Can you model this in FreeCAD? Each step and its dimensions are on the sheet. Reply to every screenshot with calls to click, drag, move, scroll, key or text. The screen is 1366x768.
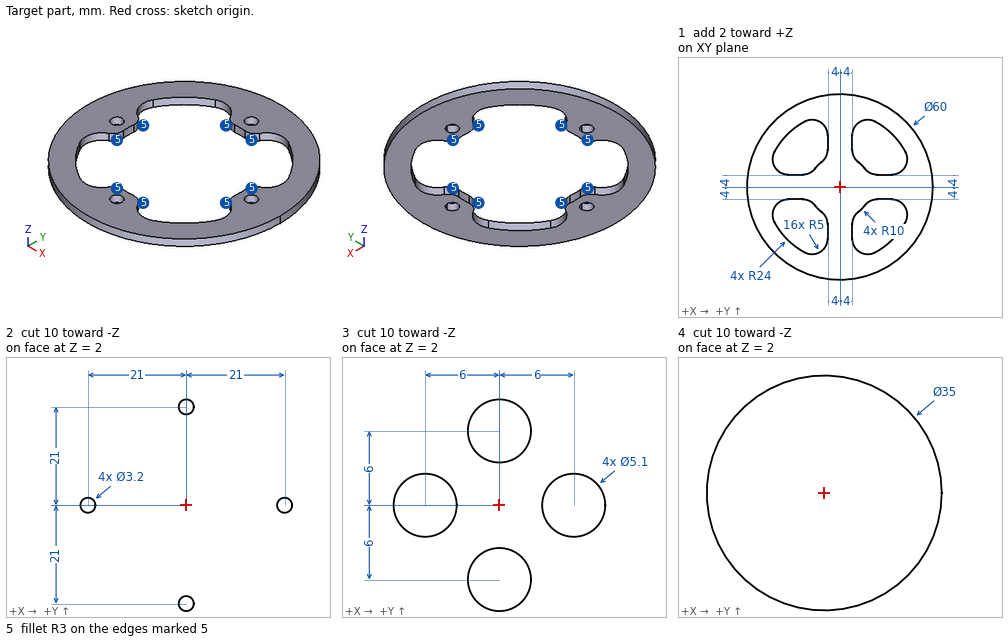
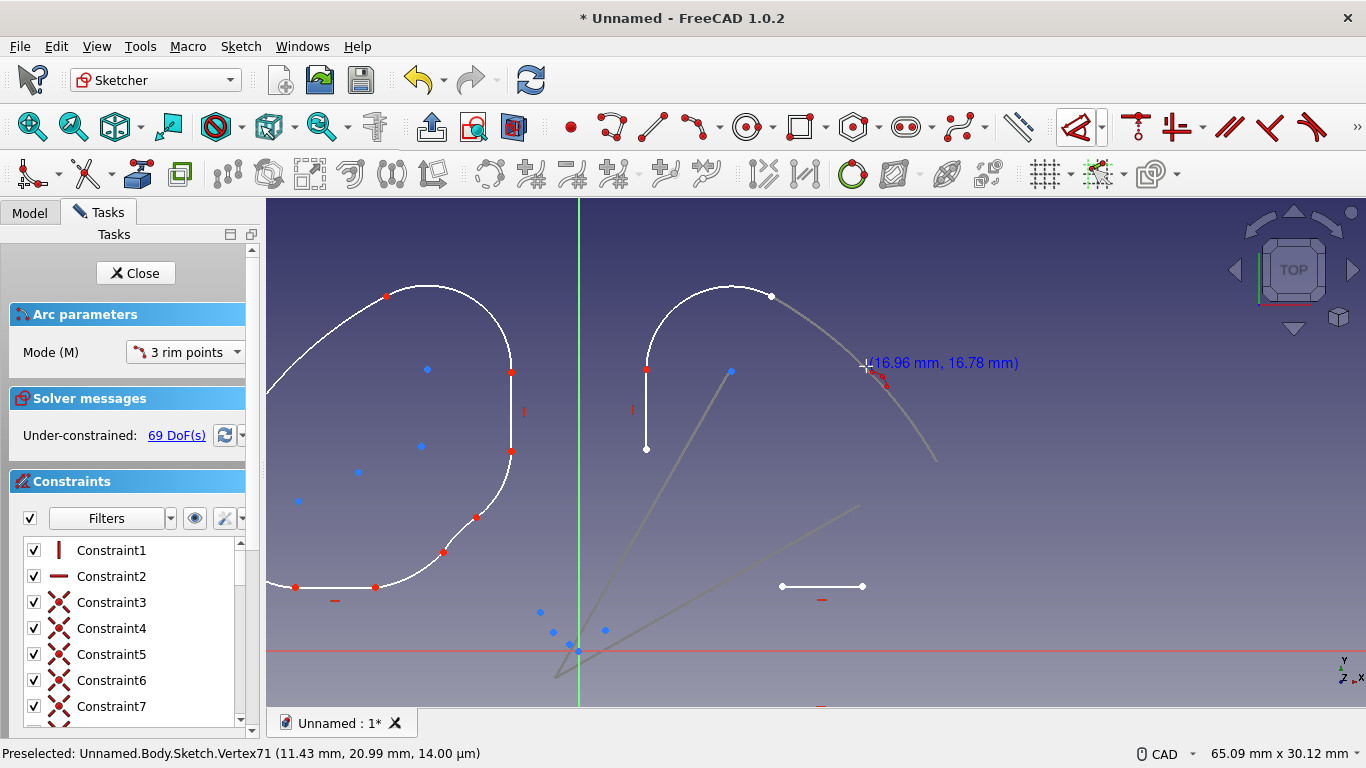
click(865, 365)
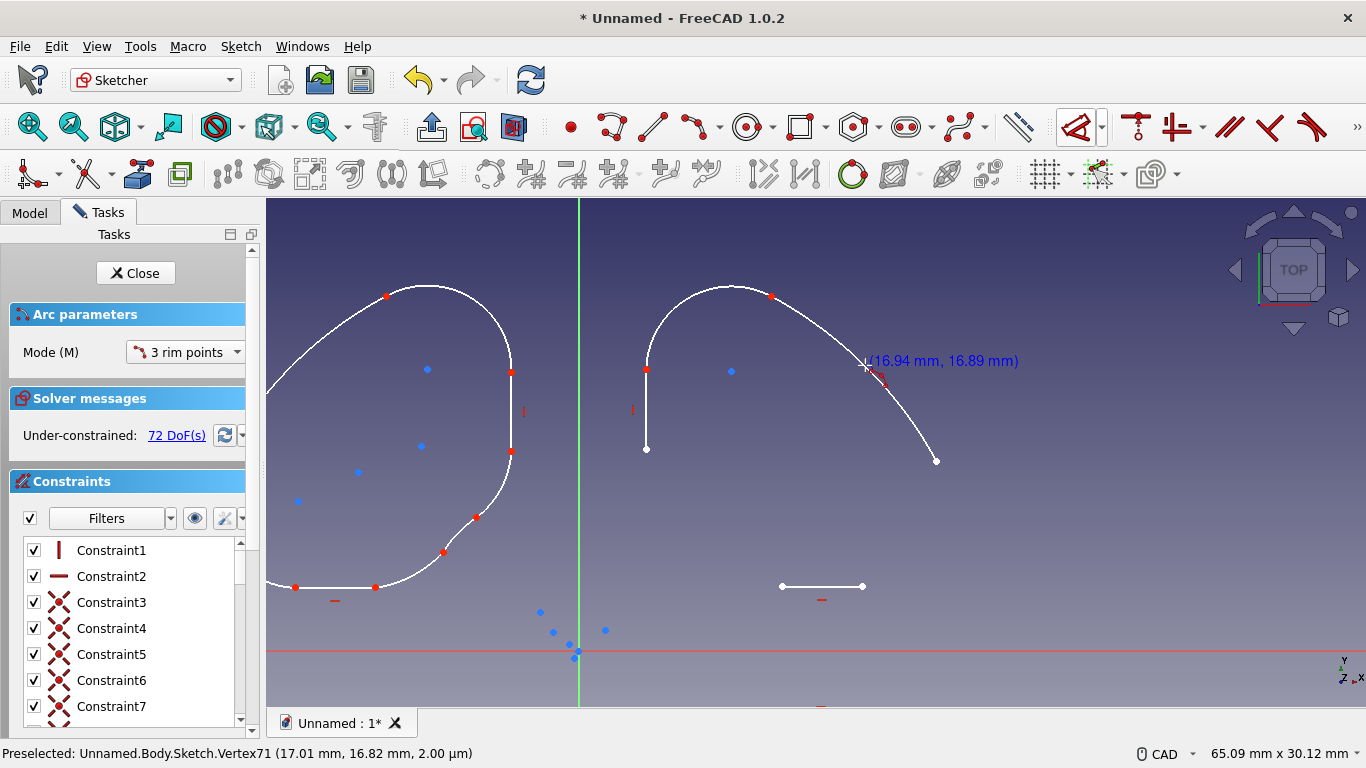
click(937, 461)
click(863, 587)
click(934, 543)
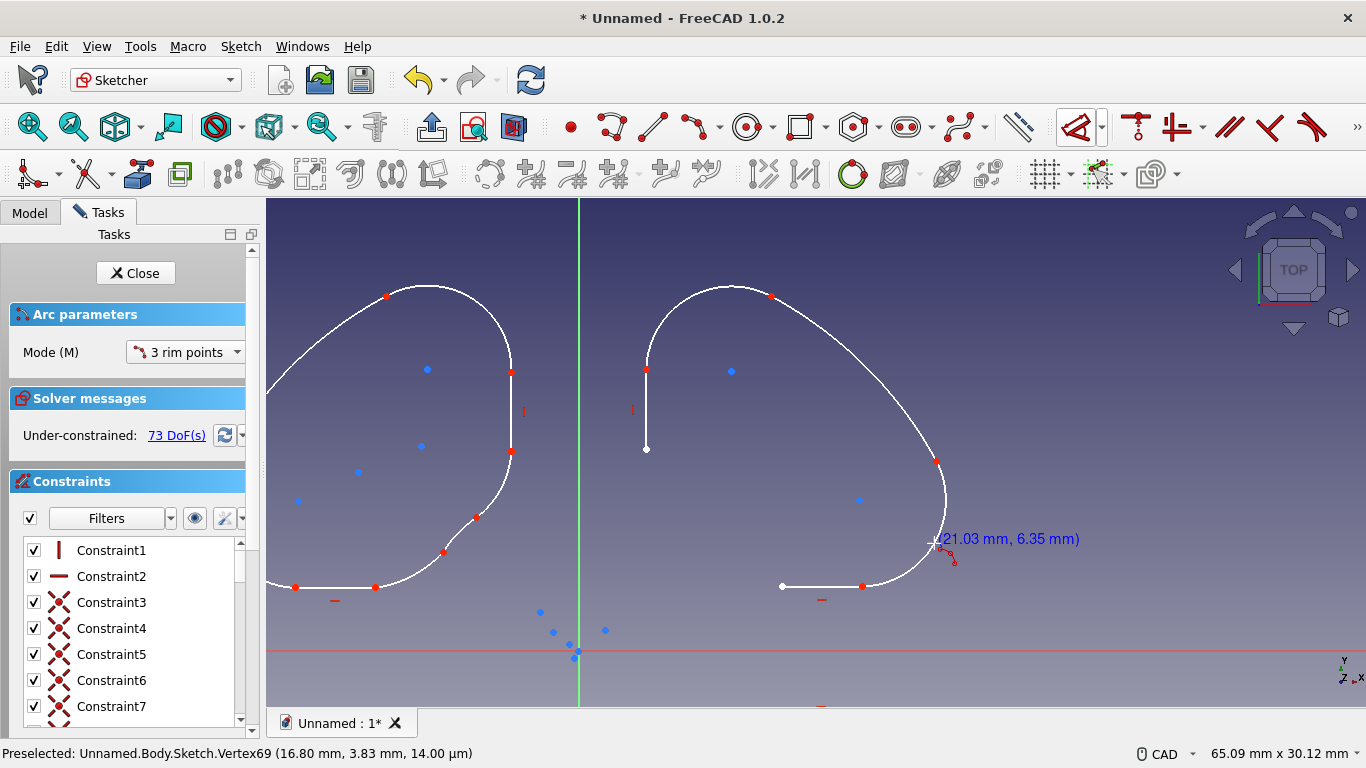
click(783, 587)
click(714, 550)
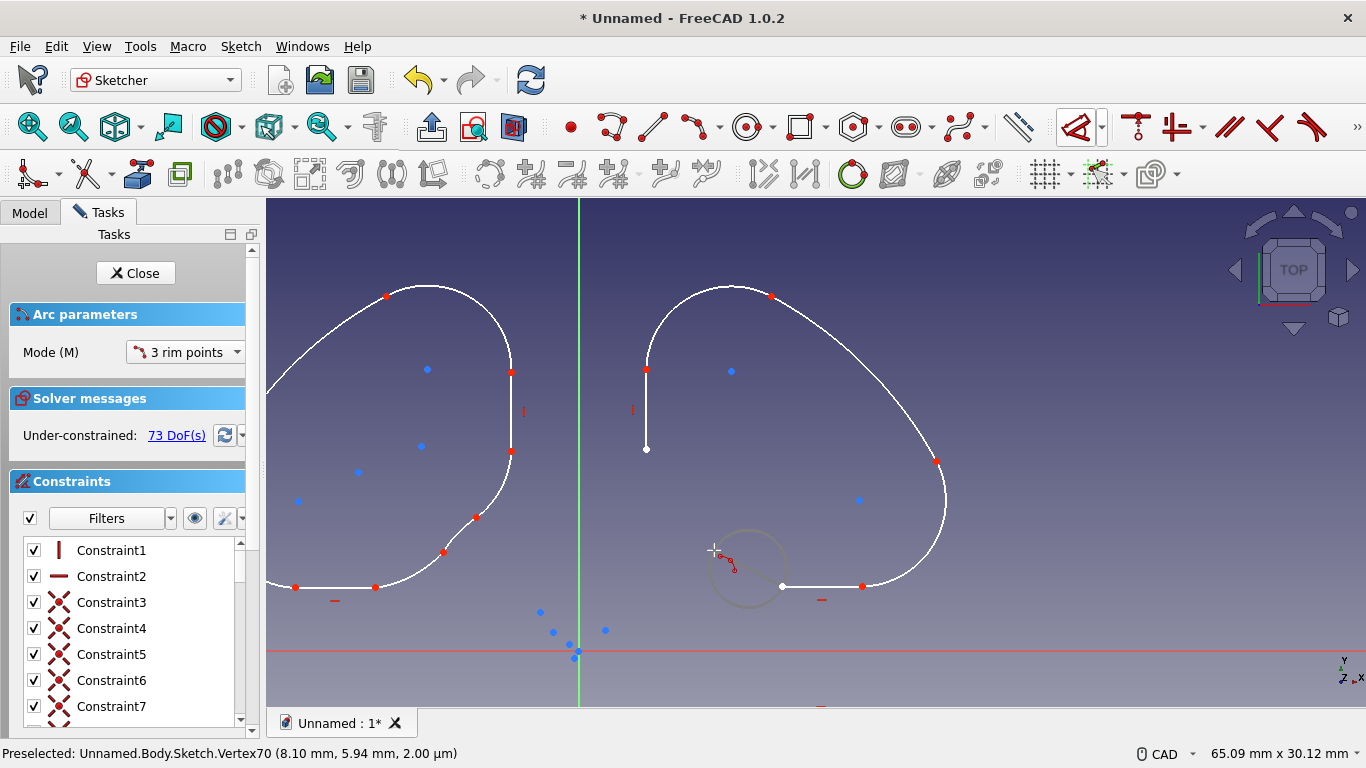
scroll(744, 575, up, 3)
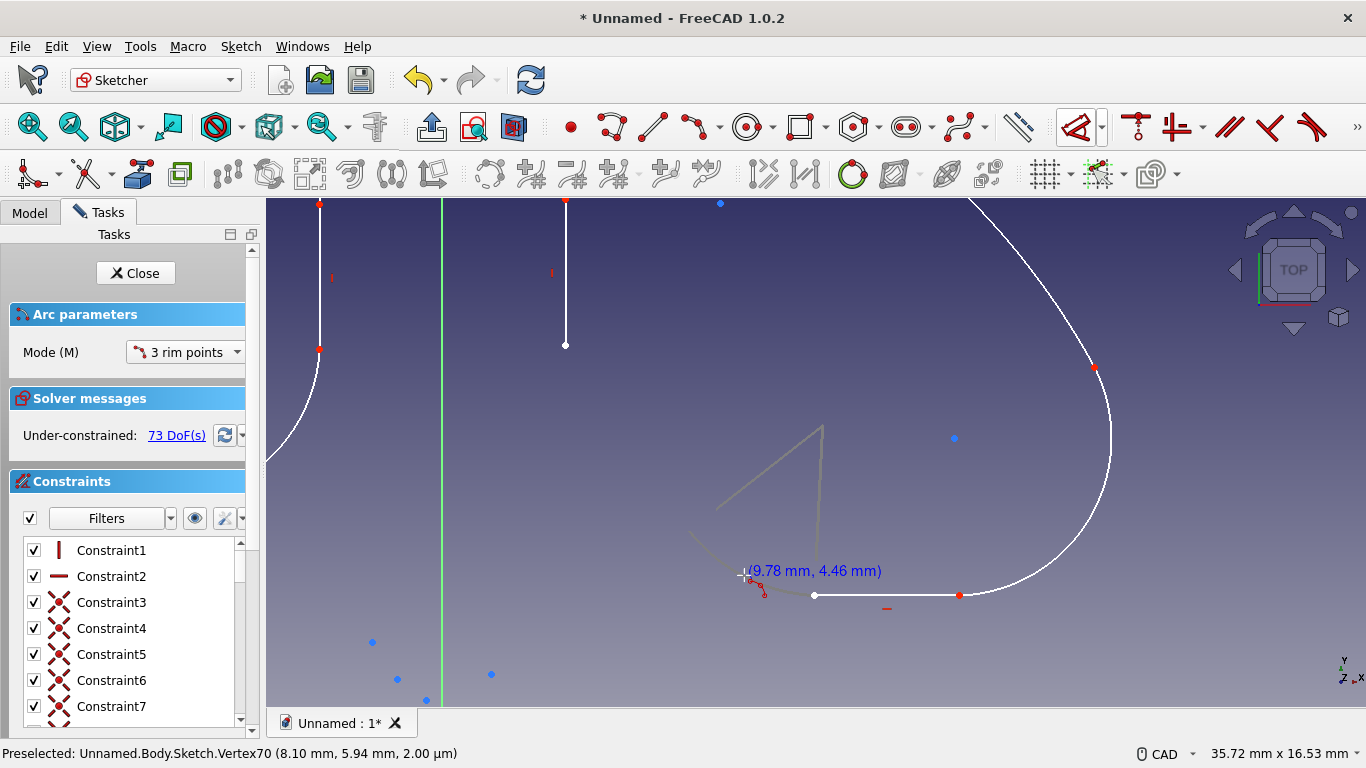
click(743, 574)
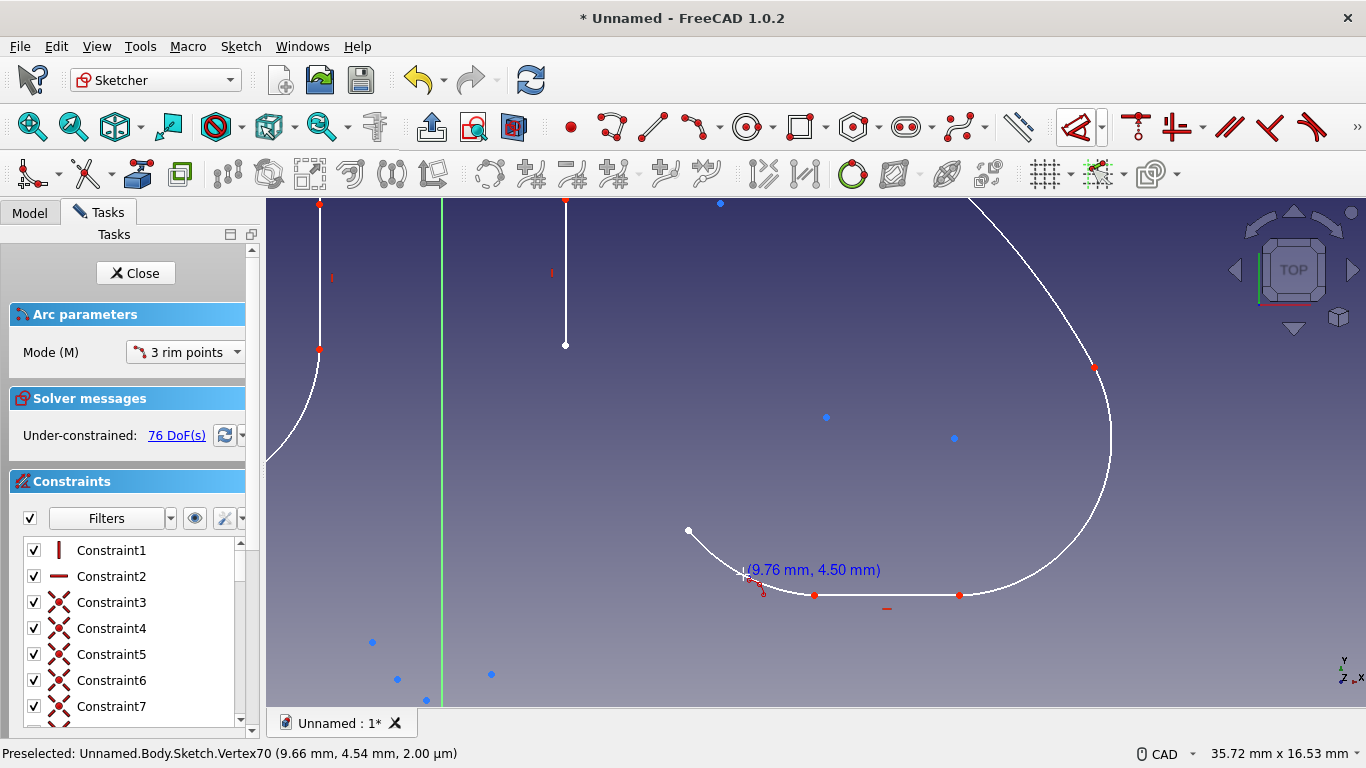
scroll(808, 401, down, 9)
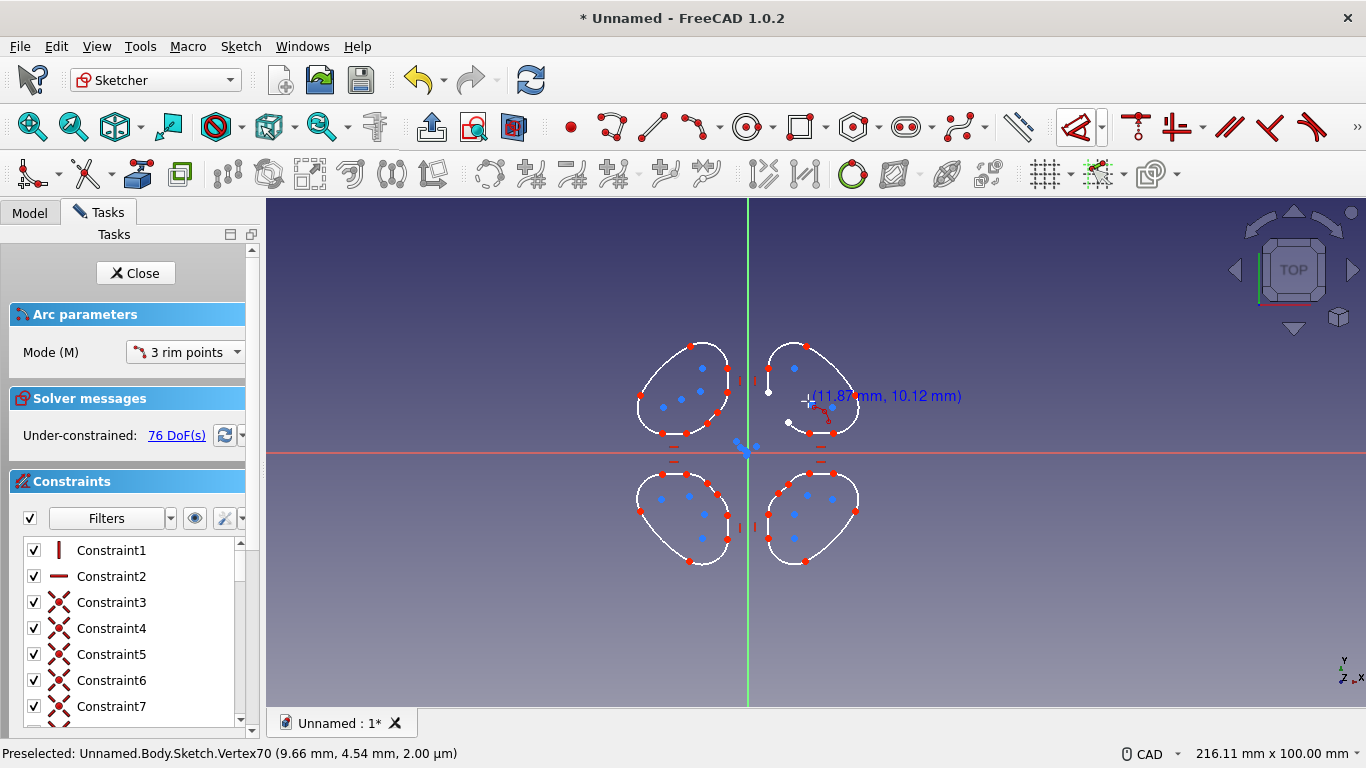
click(789, 423)
click(779, 412)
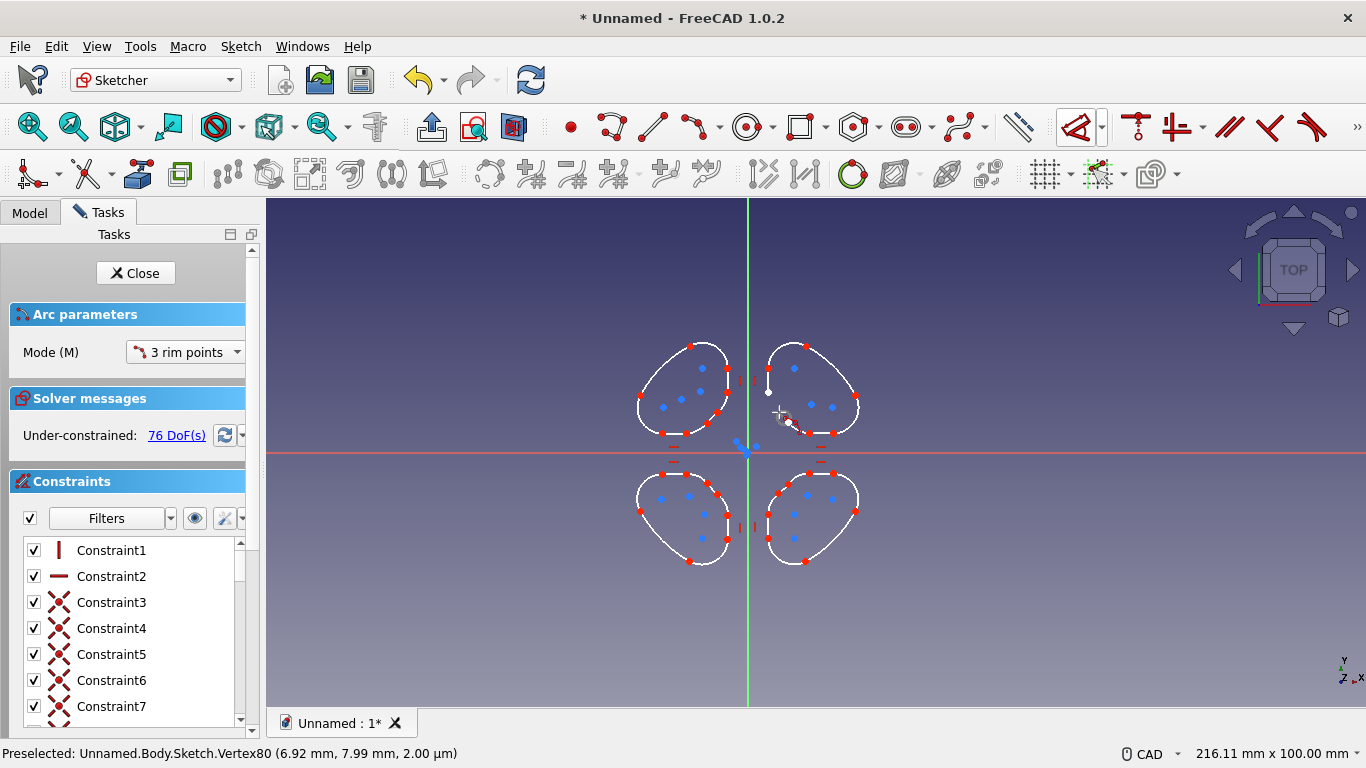
scroll(784, 417, up, 18)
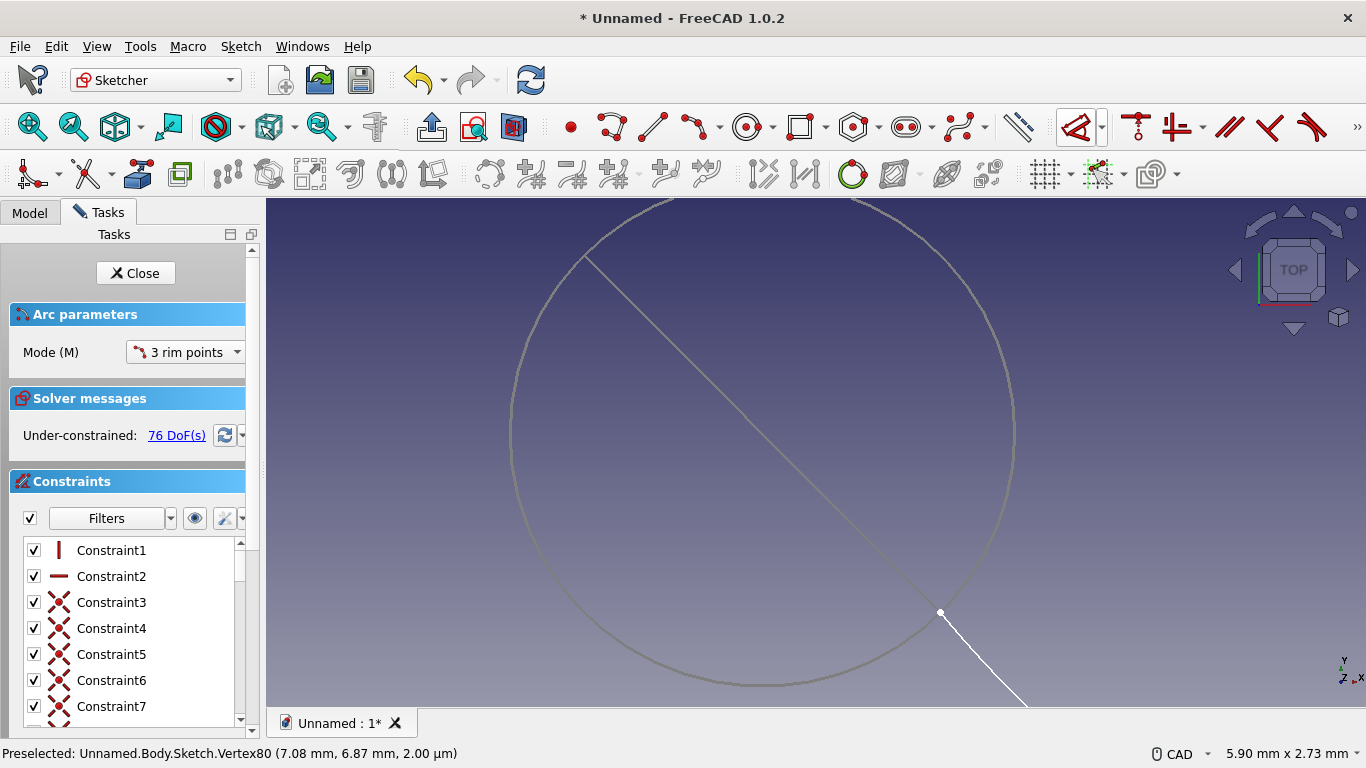
click(766, 402)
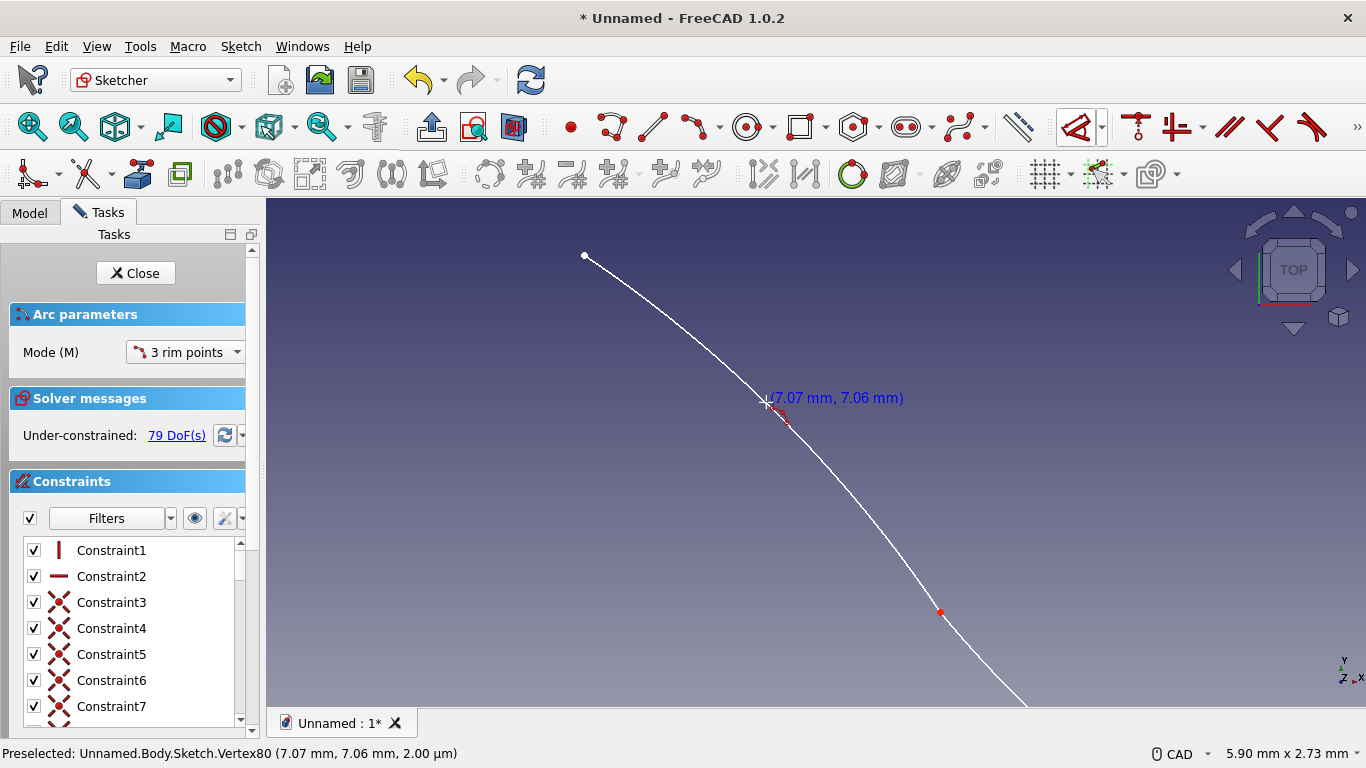
scroll(792, 409, down, 17)